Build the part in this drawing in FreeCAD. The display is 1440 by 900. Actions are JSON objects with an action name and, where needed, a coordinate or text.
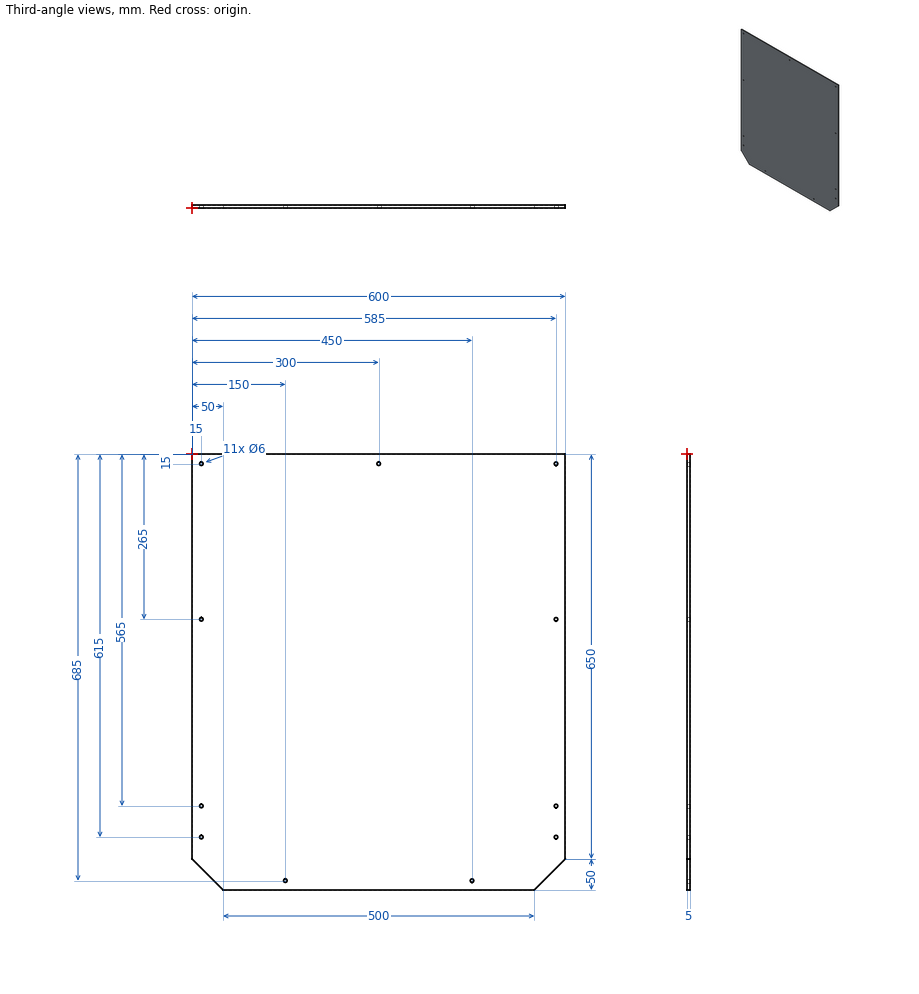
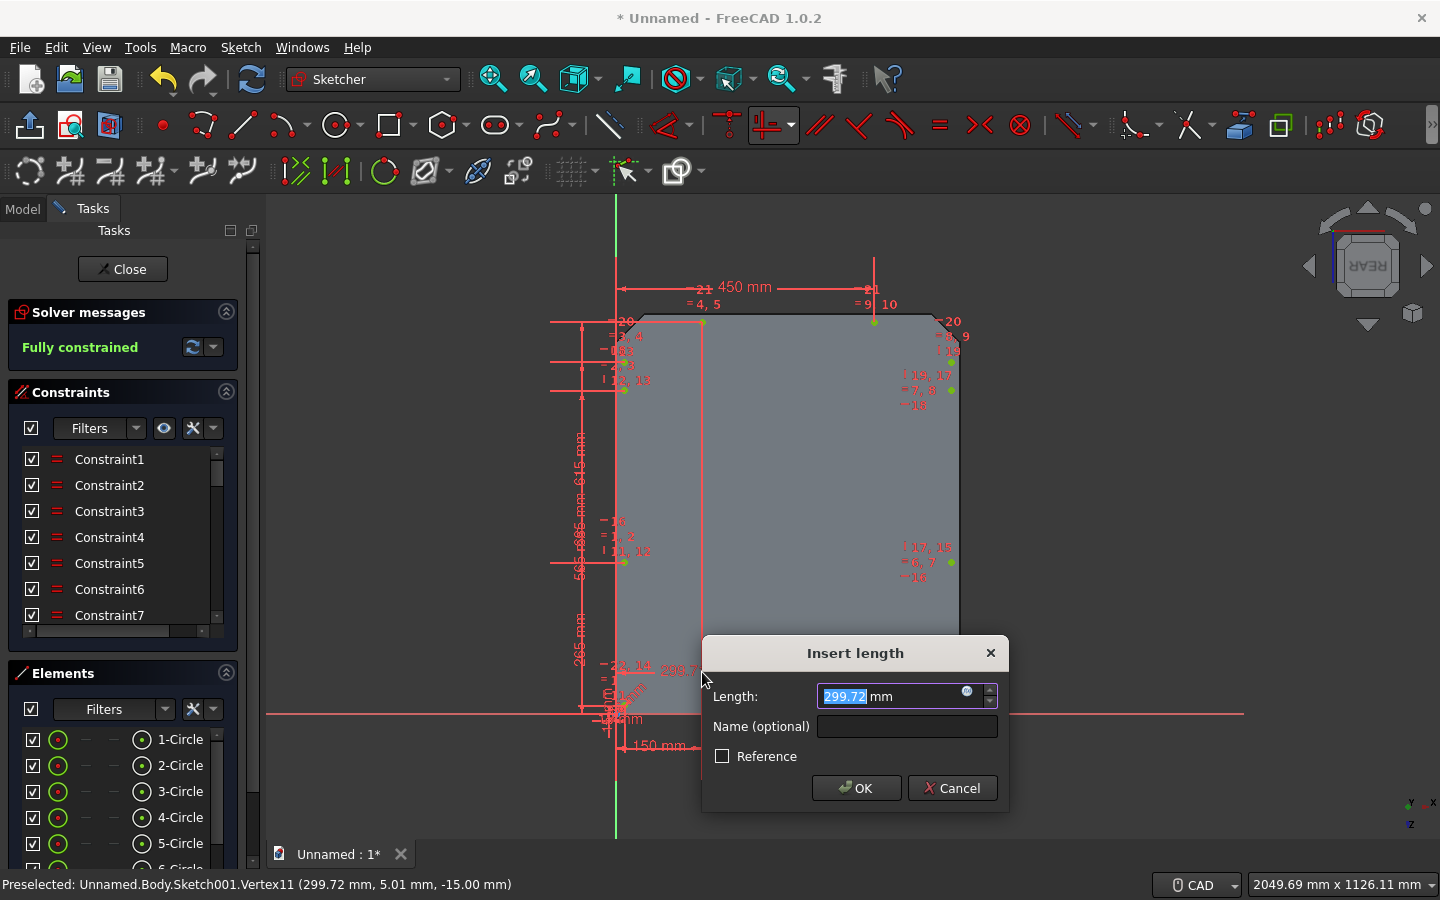
{"action": "type", "text": "300"}
{"action": "key", "text": "Return"}
{"action": "key", "text": "Escape"}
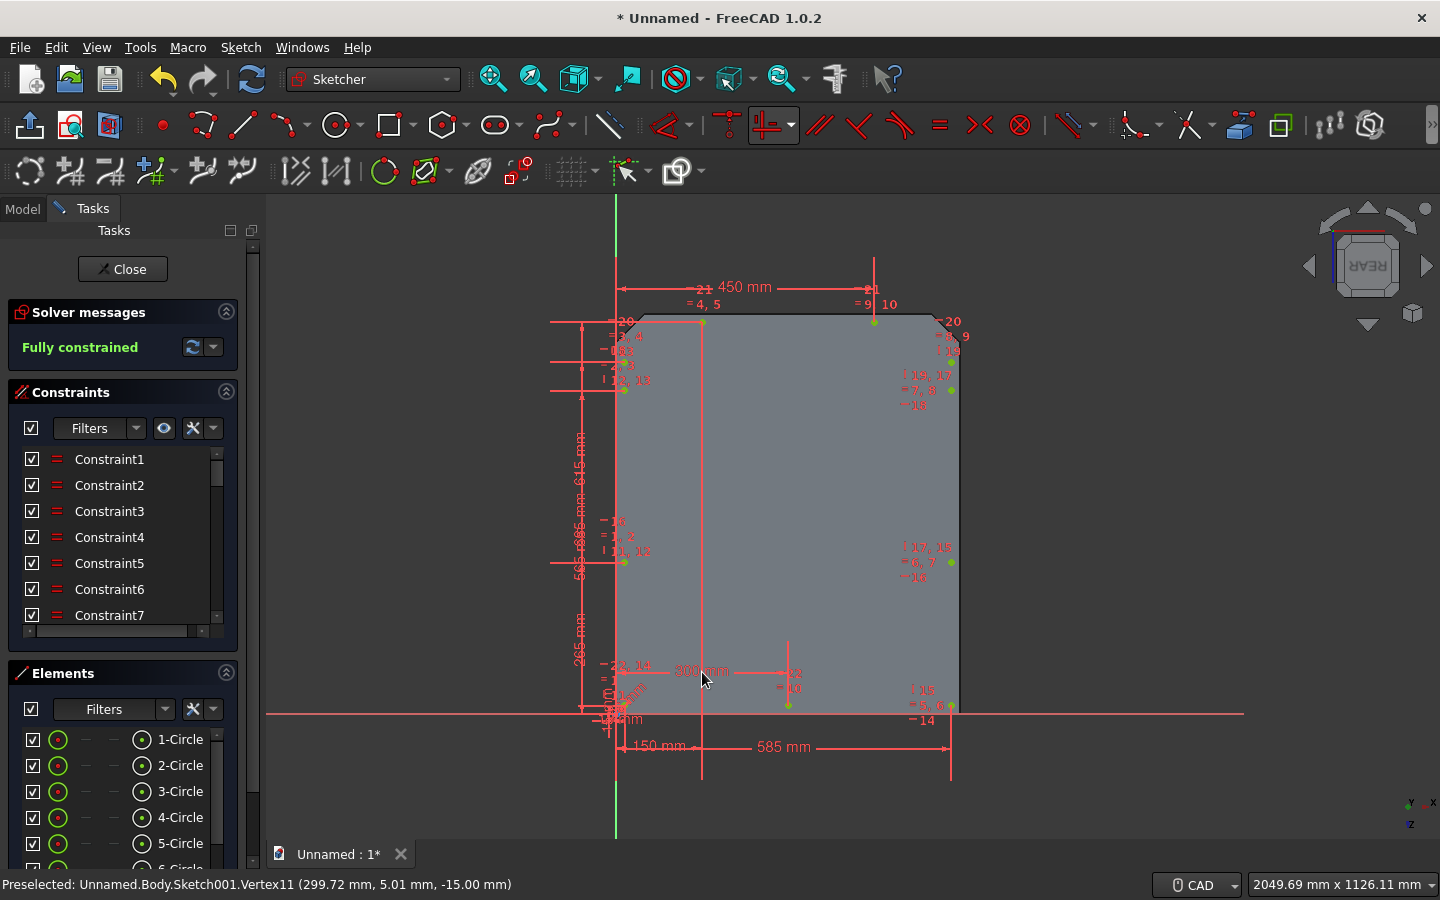
{"action": "left_click", "coordinate": [123, 269]}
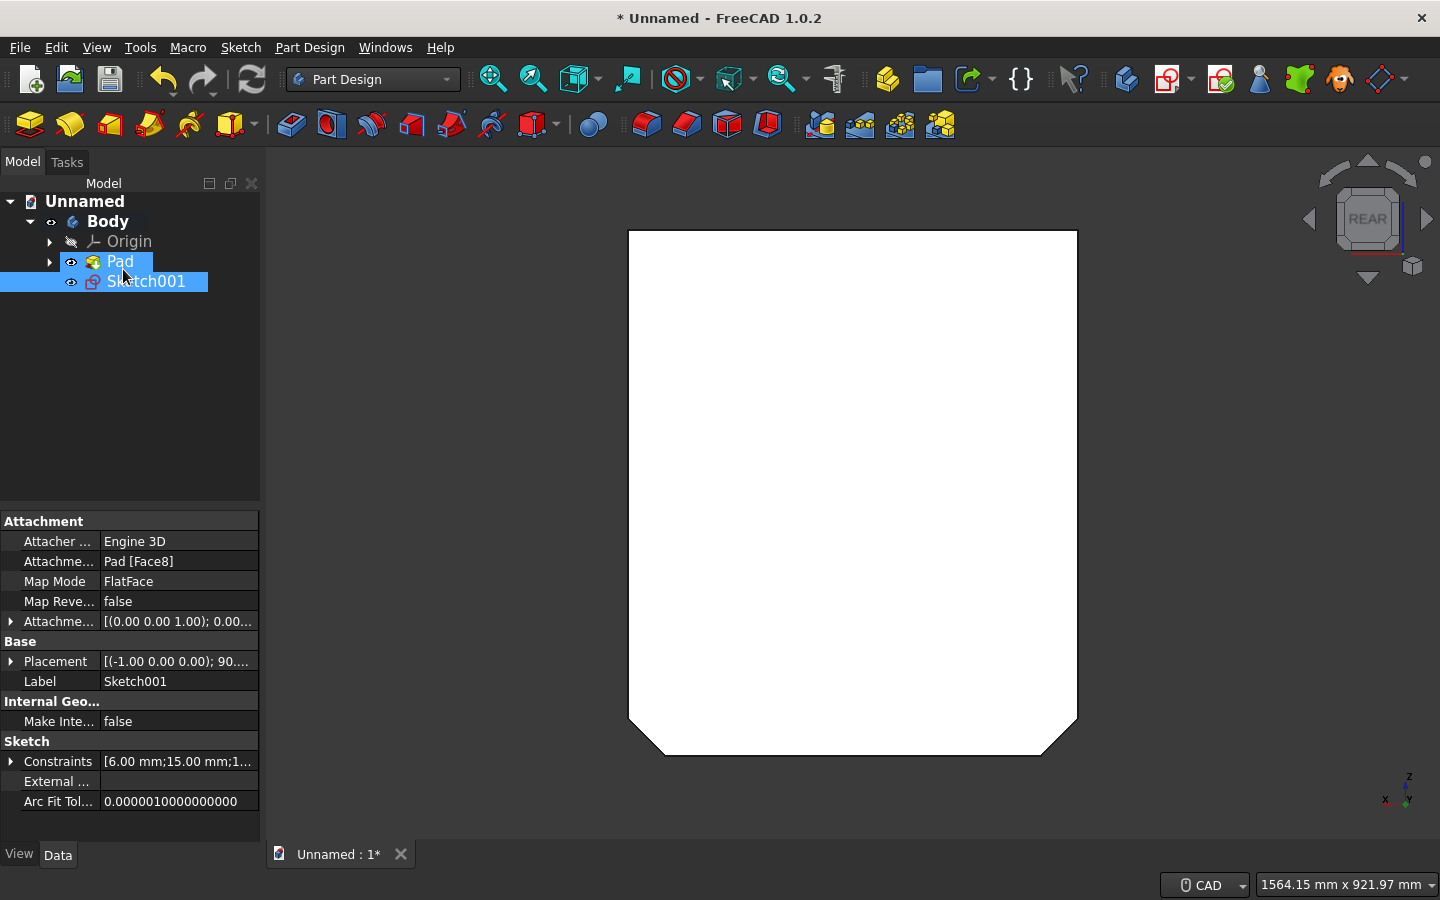
{"action": "left_click", "coordinate": [292, 124]}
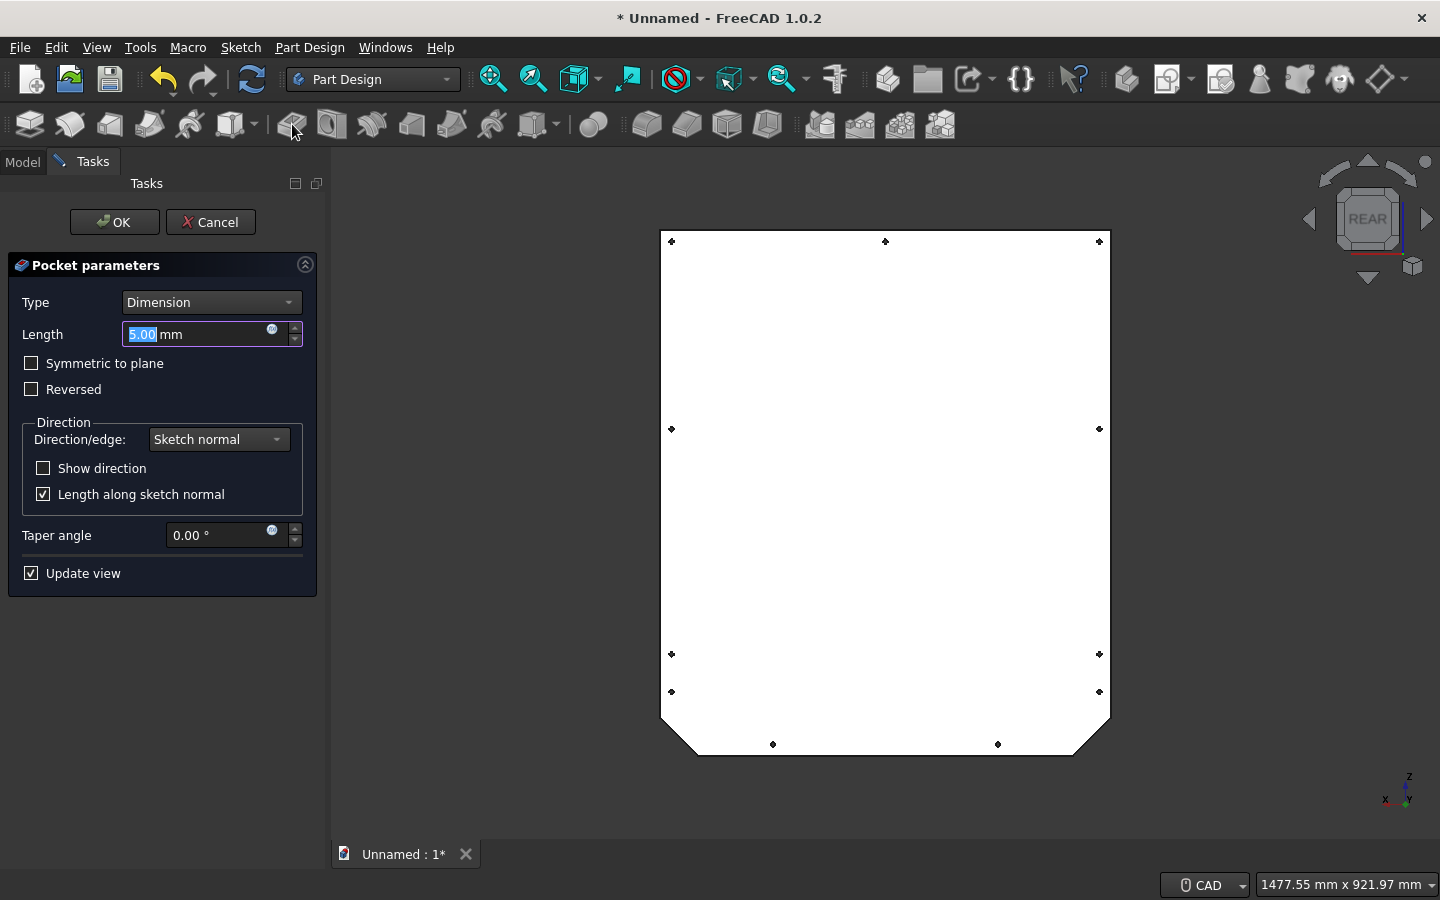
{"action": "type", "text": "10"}
{"action": "key", "text": "Tab"}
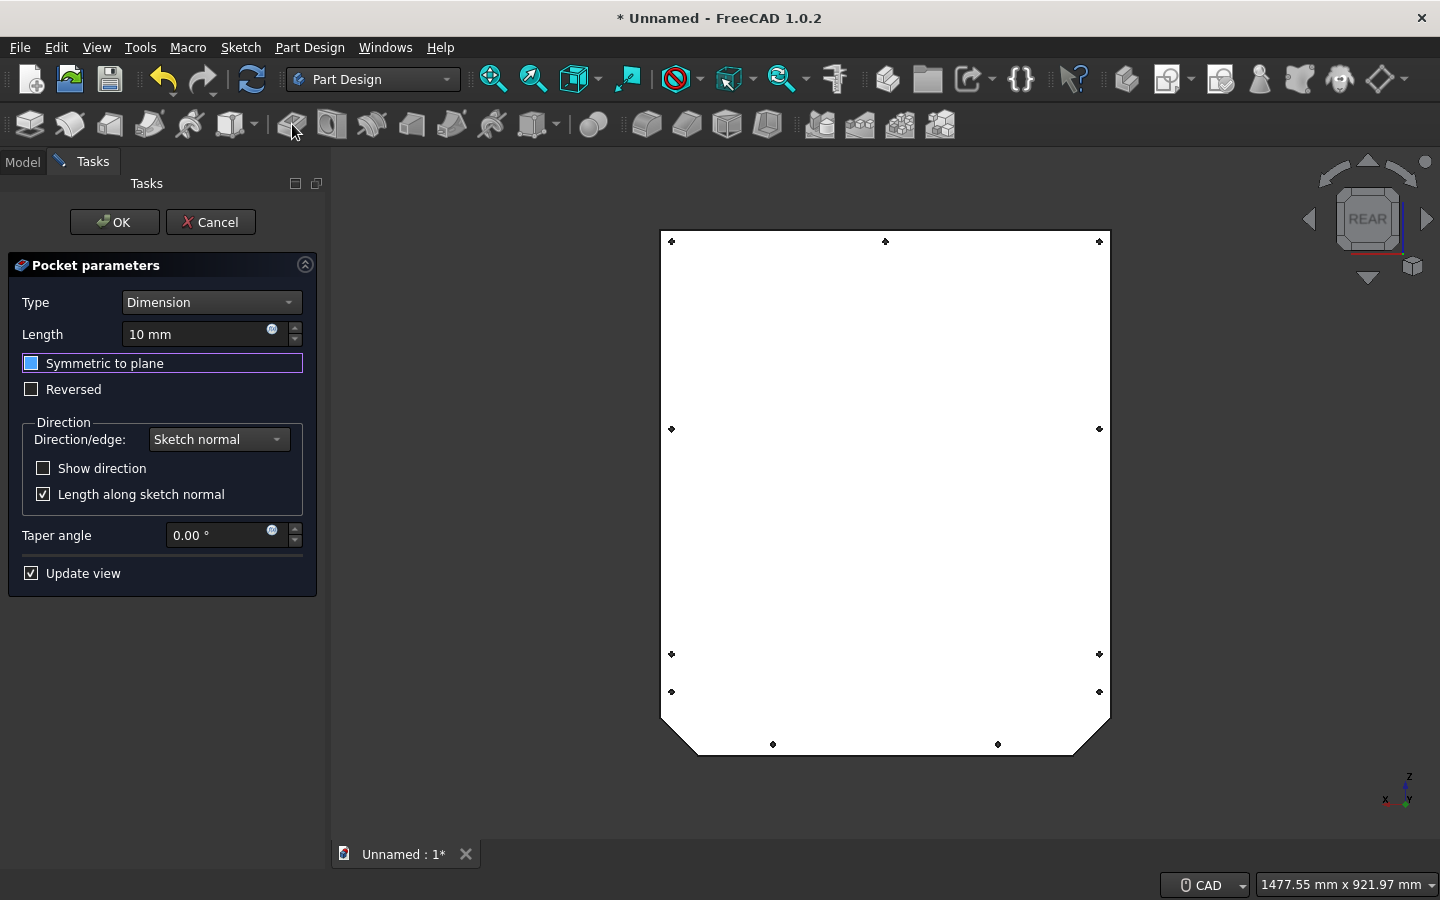
{"action": "left_click", "coordinate": [115, 222]}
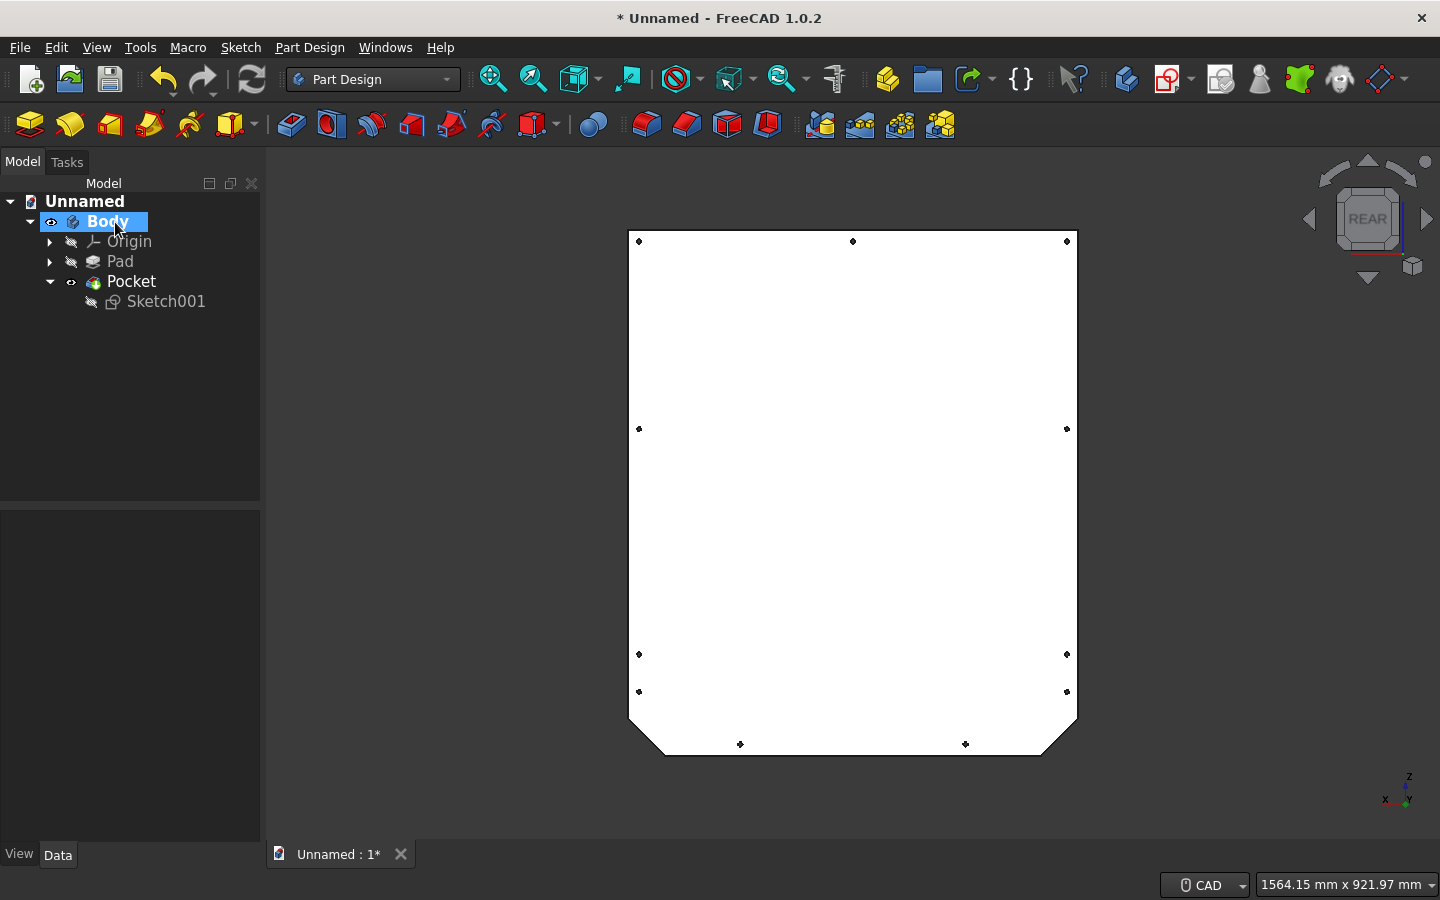
{"action": "key", "text": "0"}